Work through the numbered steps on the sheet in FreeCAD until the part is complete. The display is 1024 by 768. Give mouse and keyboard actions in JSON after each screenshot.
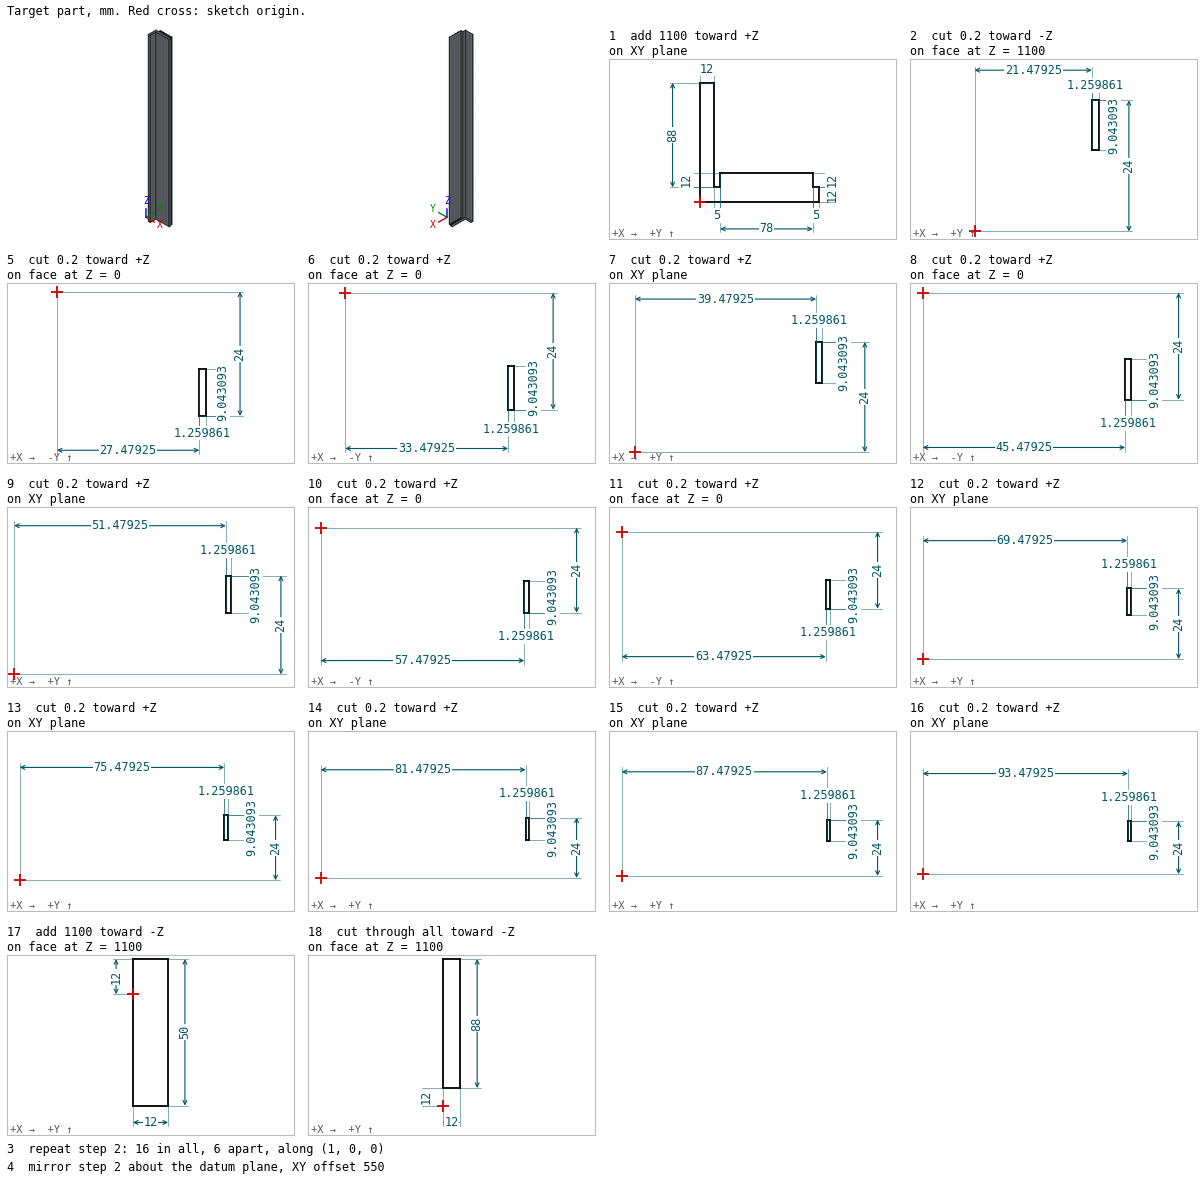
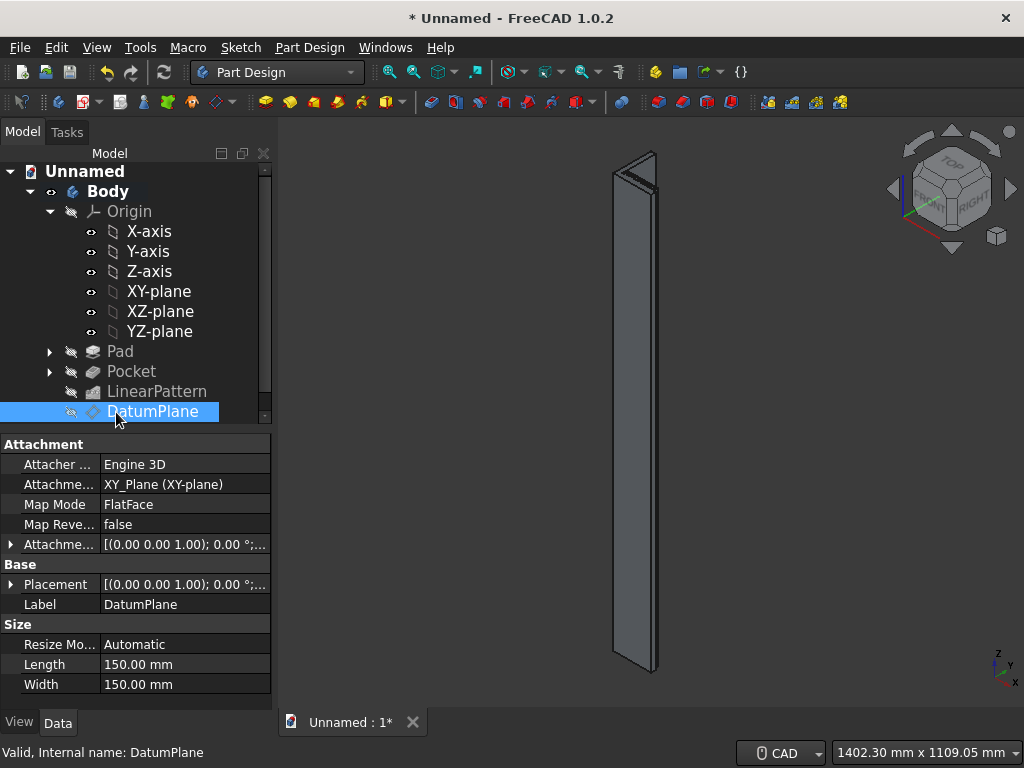
{"action": "key", "text": "5"}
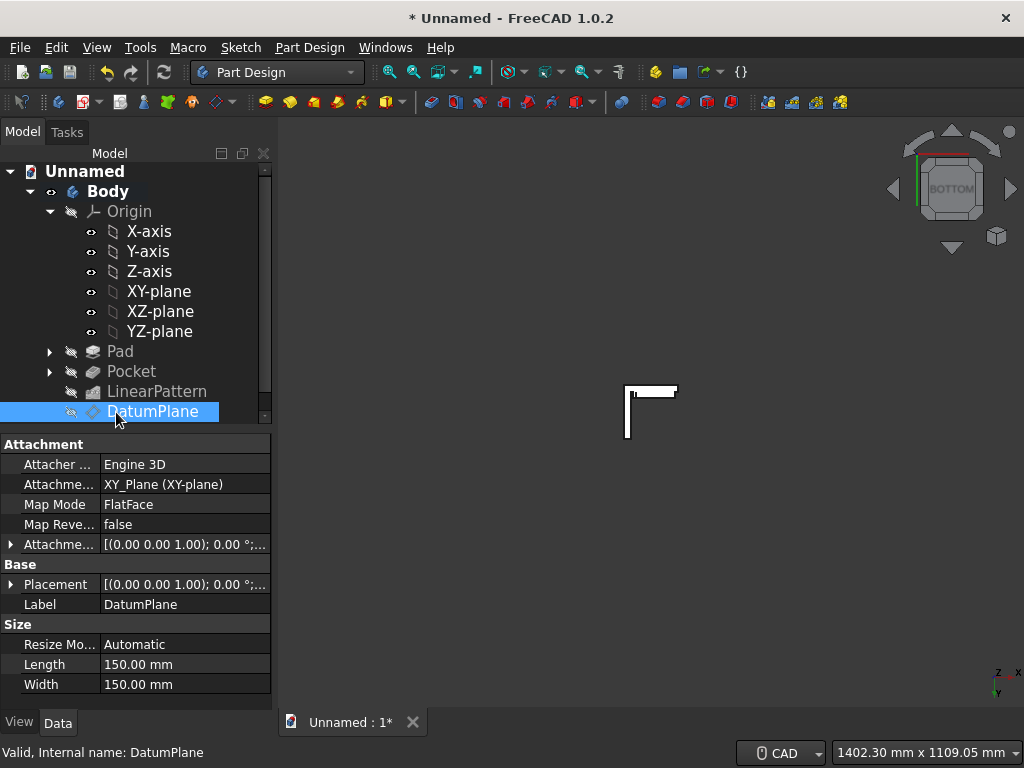
{"action": "key", "text": "v f"}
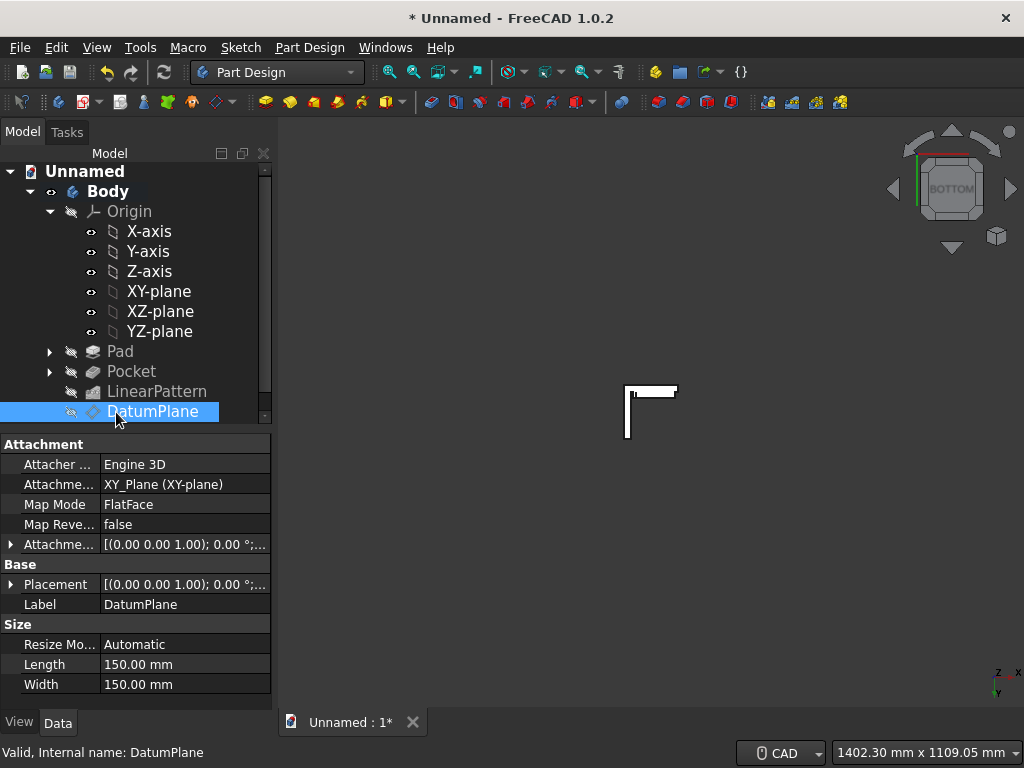
{"action": "scroll", "coordinate": [666, 388], "scroll_direction": "up", "scroll_amount": 6}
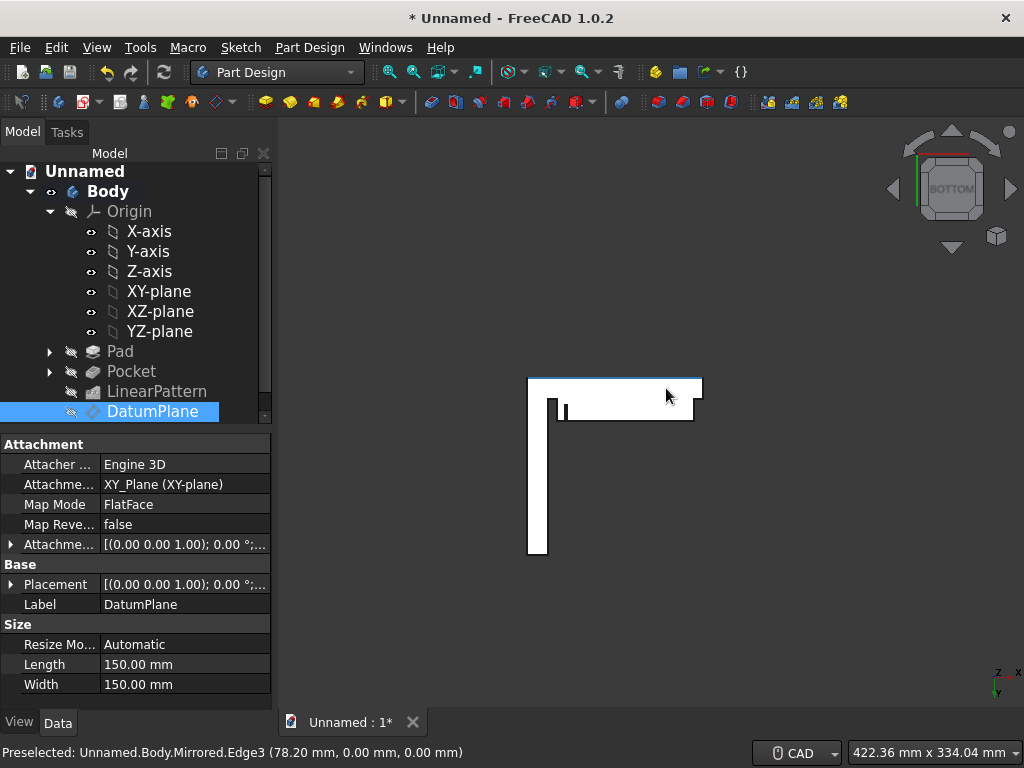
{"action": "left_click", "coordinate": [665, 390]}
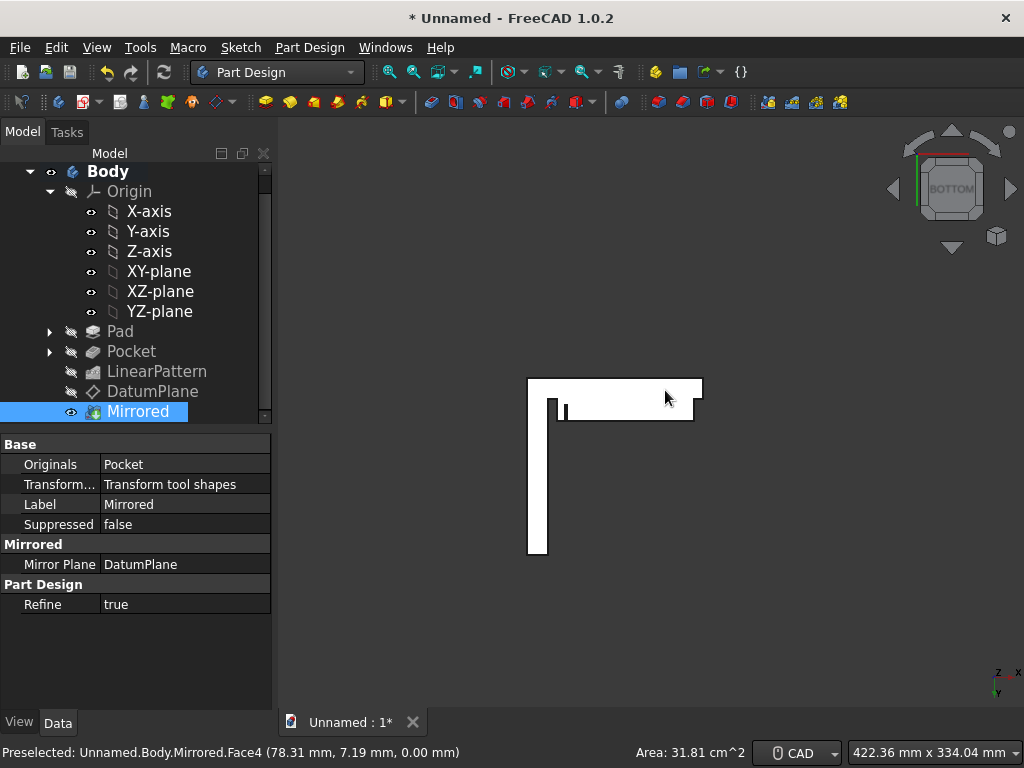
{"action": "left_click", "coordinate": [84, 102]}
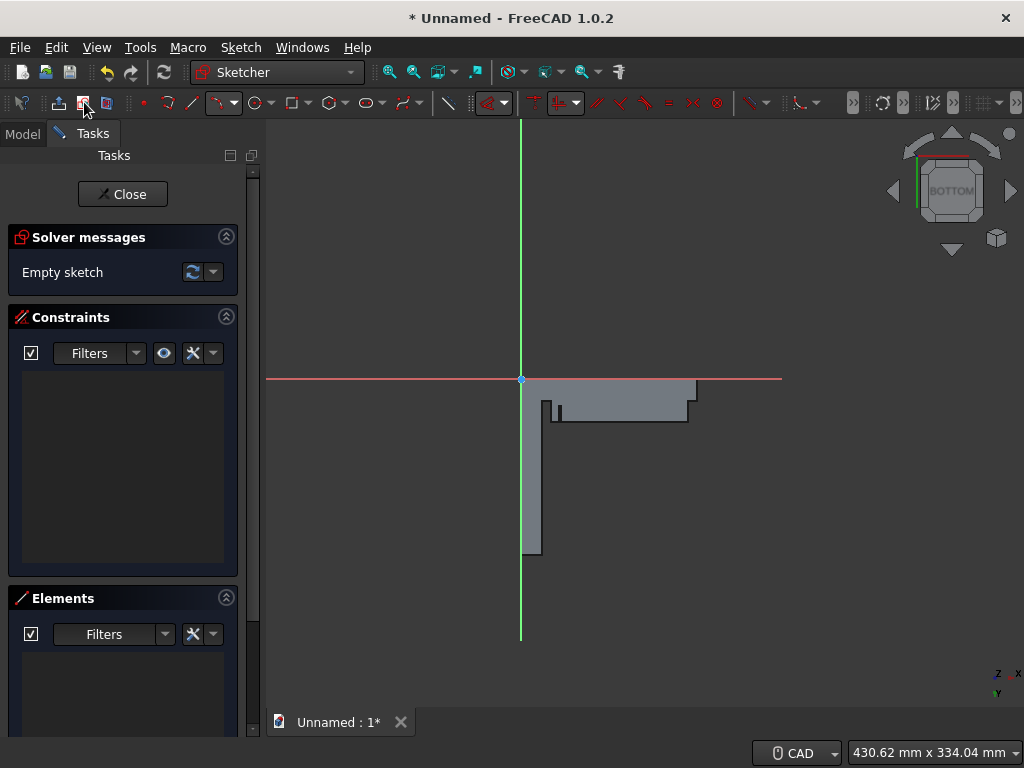
{"action": "scroll", "coordinate": [570, 414], "scroll_direction": "up", "scroll_amount": 15}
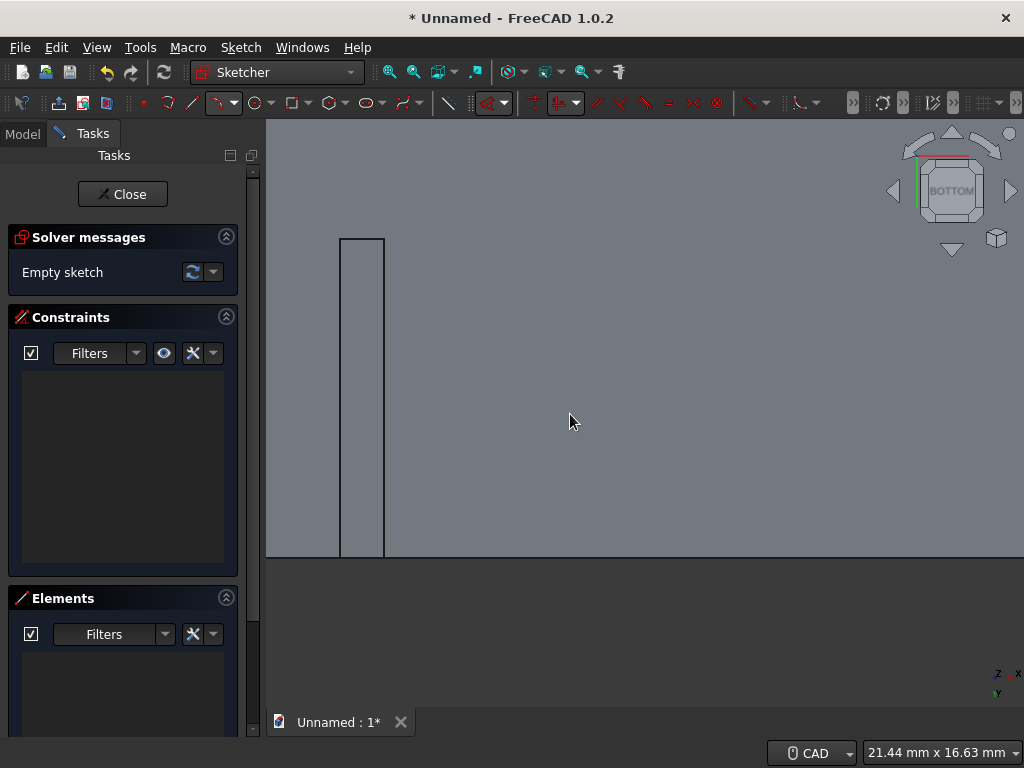
{"action": "key", "text": "g r"}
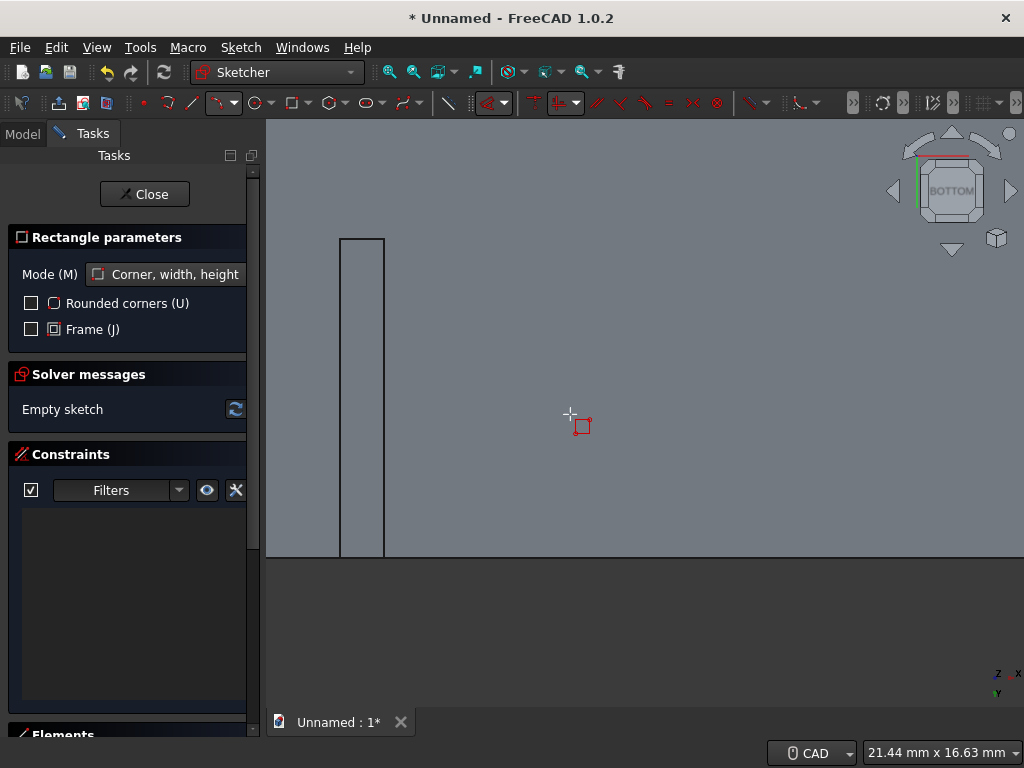
{"action": "left_click", "coordinate": [552, 239]}
{"action": "mouse_move", "coordinate": [596, 558]}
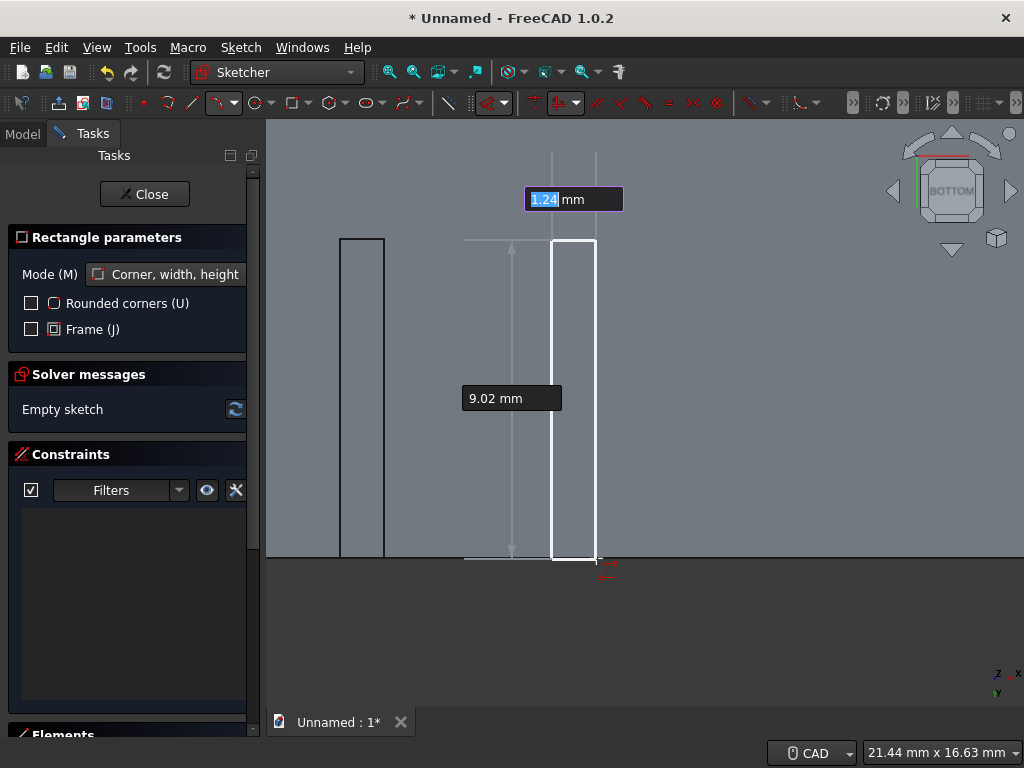
{"action": "type", "text": "1.259861"}
{"action": "key", "text": "Tab"}
{"action": "type", "text": "9.043093"}
{"action": "key", "text": "Return"}
{"action": "key", "text": "Escape"}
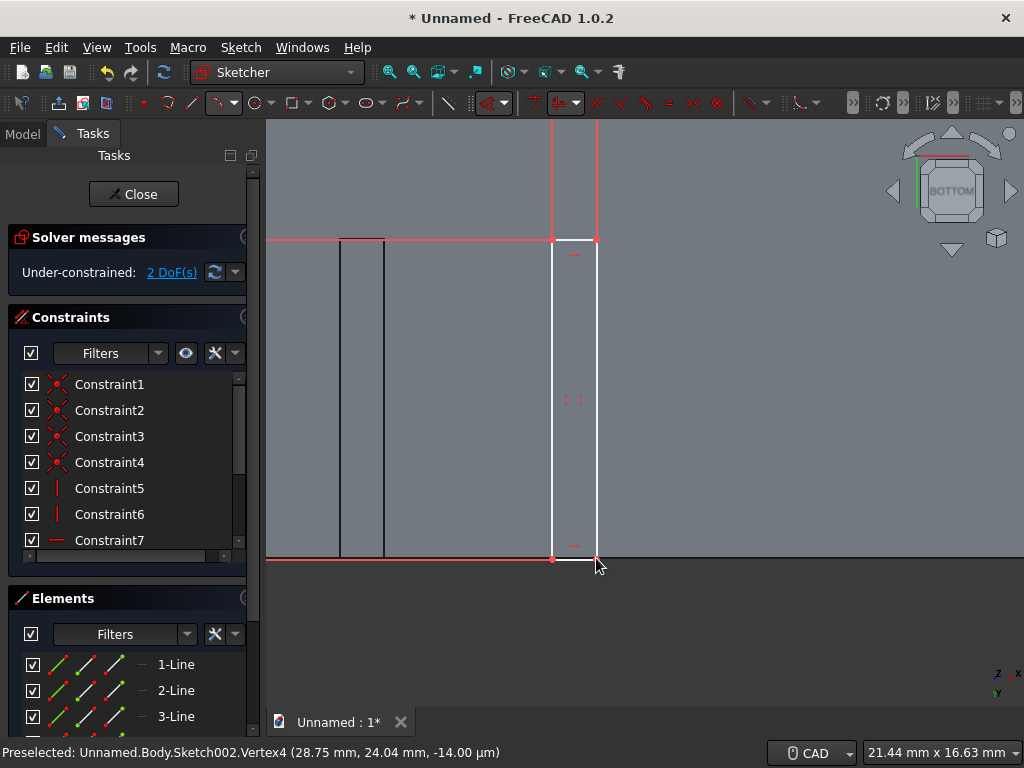
{"action": "left_click", "coordinate": [552, 560]}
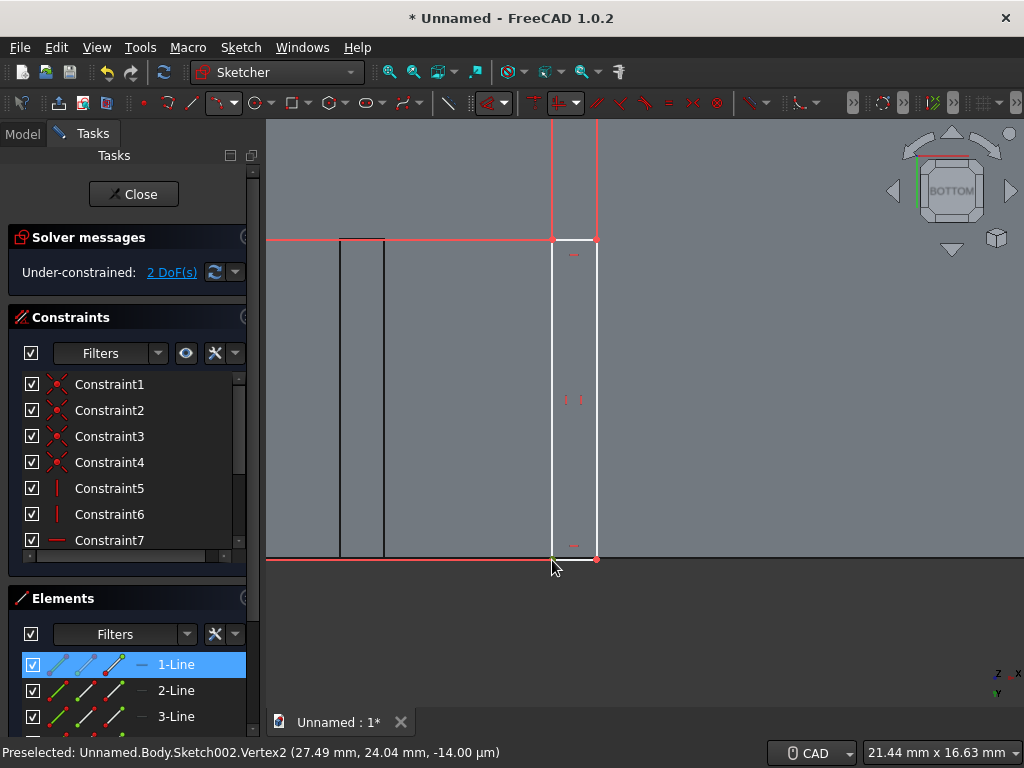
{"action": "left_click", "coordinate": [506, 104]}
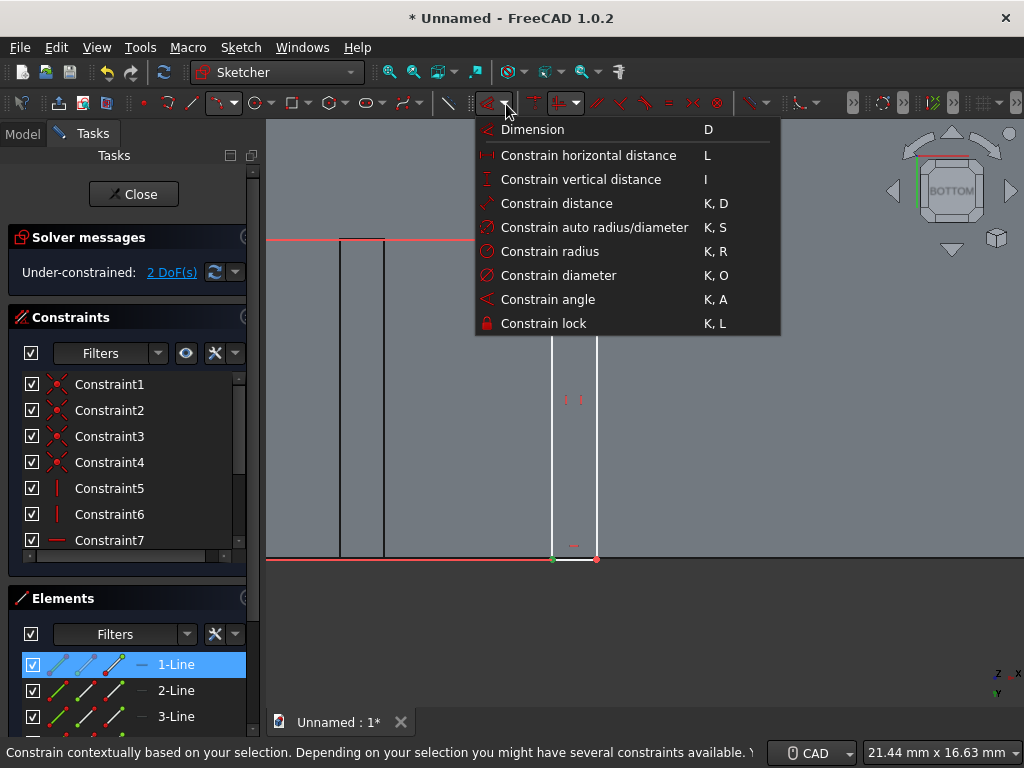
{"action": "left_click", "coordinate": [628, 179]}